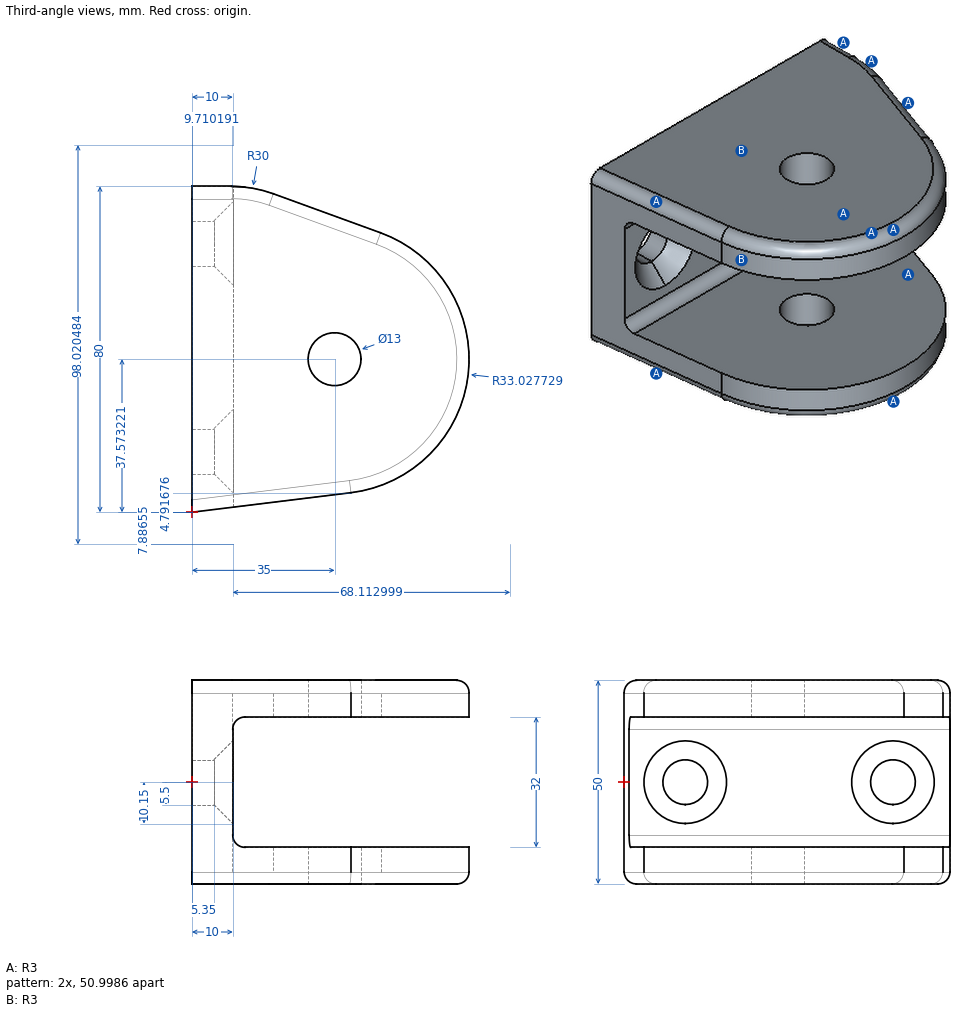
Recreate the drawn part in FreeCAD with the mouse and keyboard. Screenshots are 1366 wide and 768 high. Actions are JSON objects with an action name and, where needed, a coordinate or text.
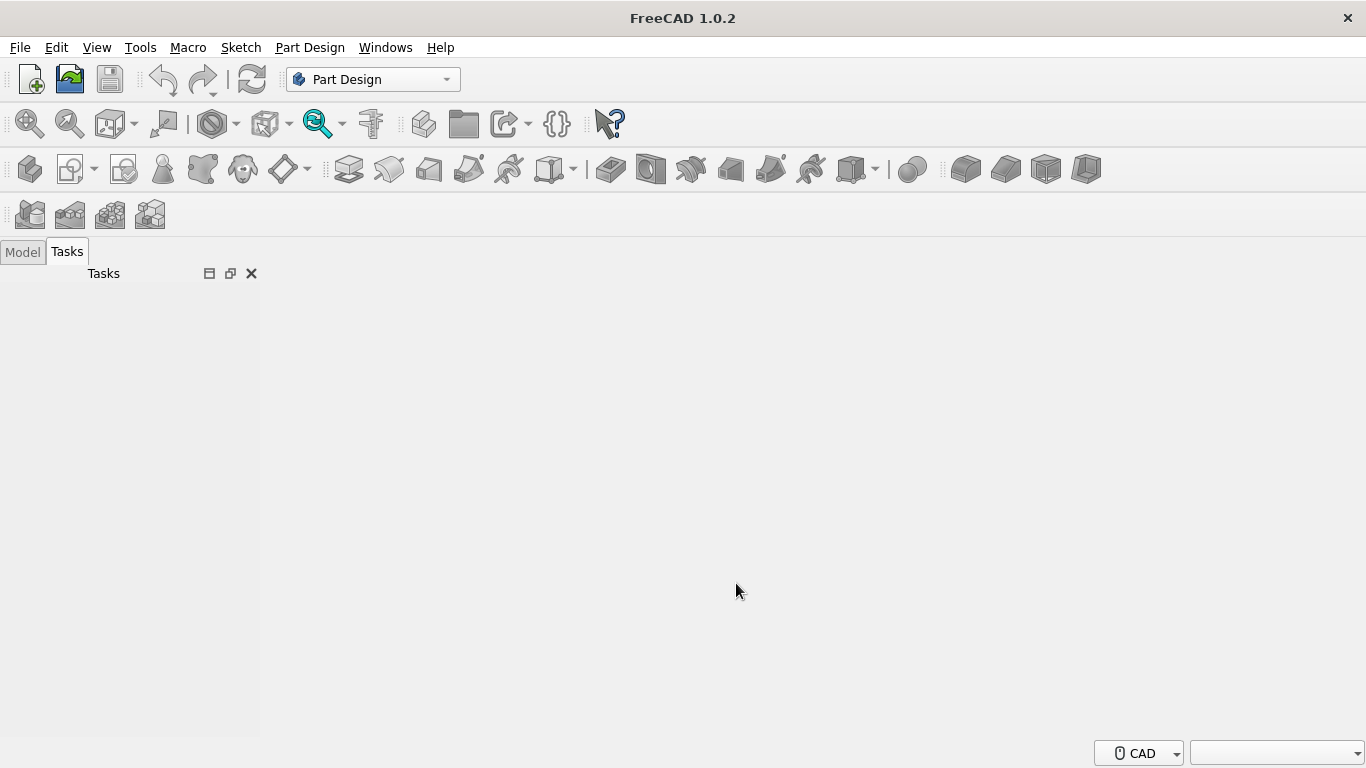
{"action": "left_click", "coordinate": [30, 80]}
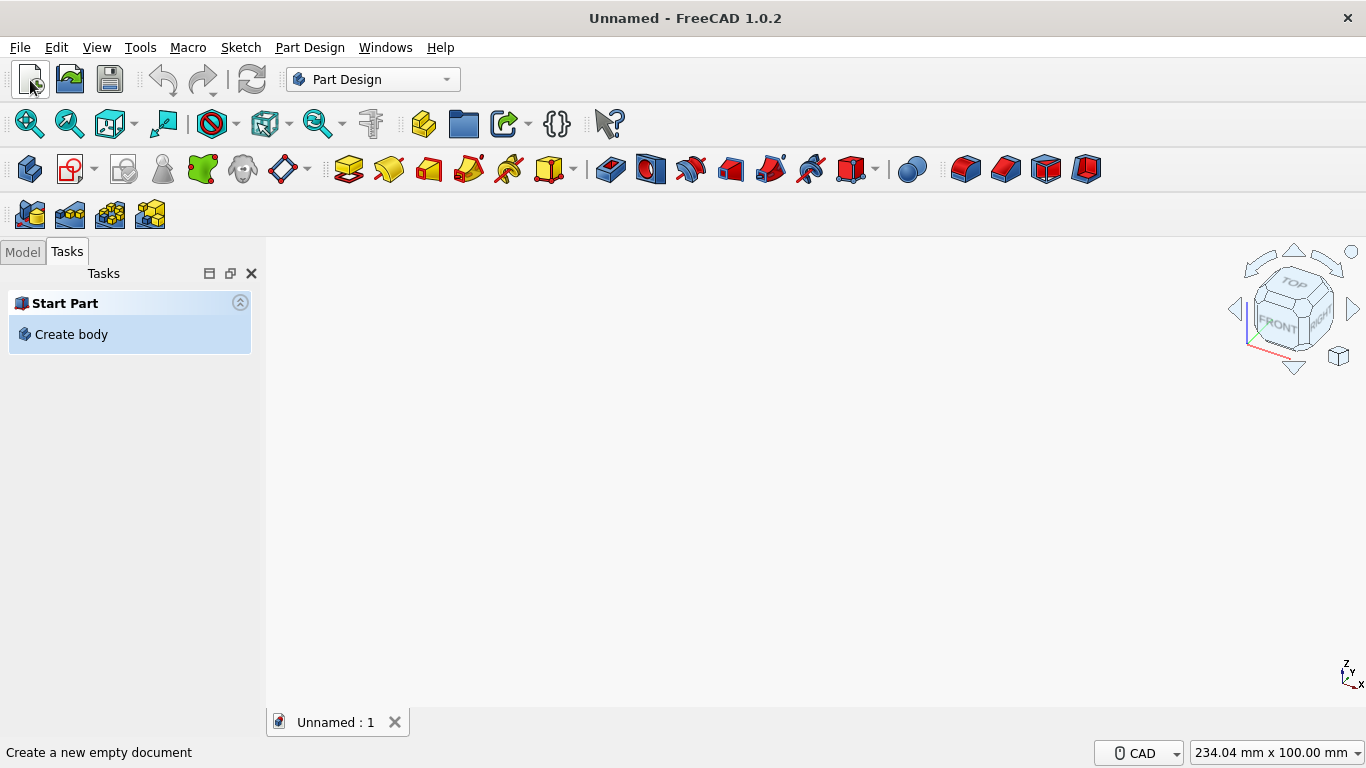
{"action": "left_click", "coordinate": [70, 170]}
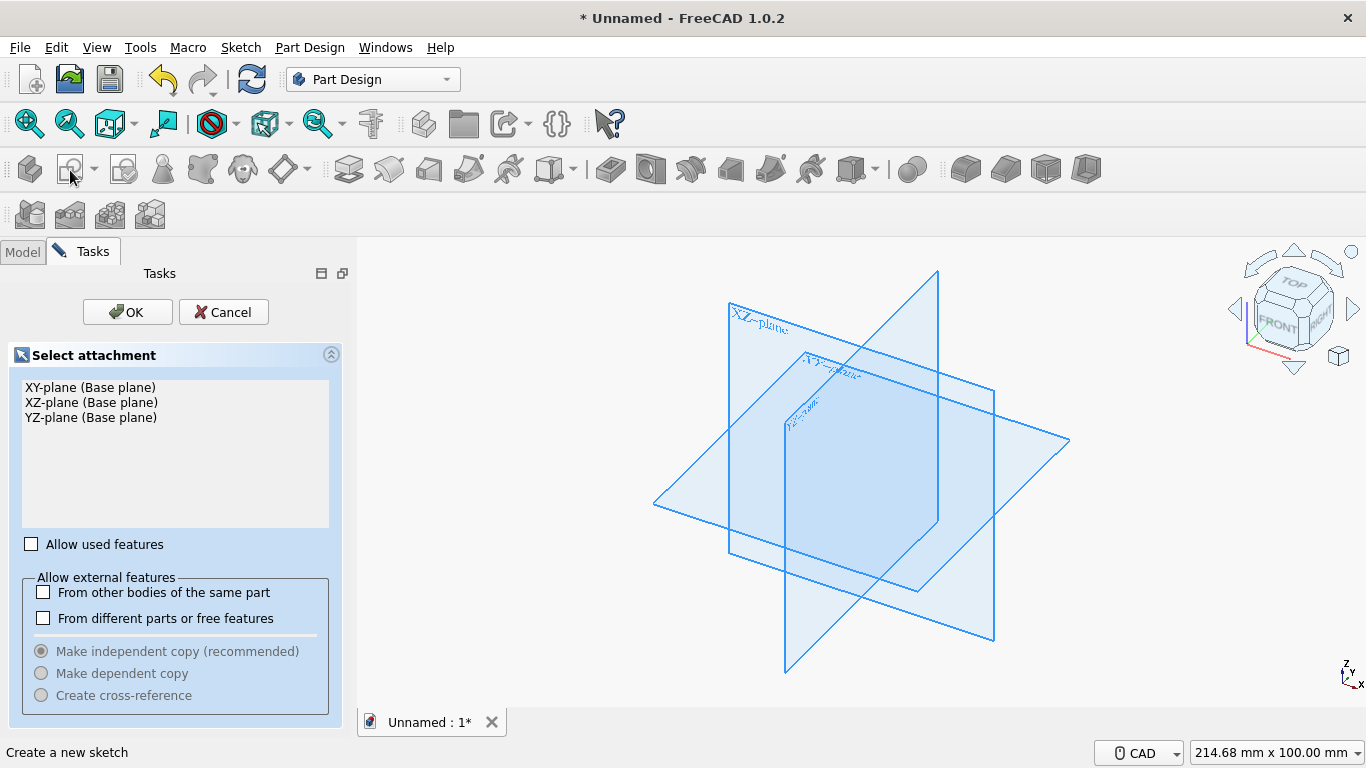
{"action": "left_click", "coordinate": [82, 388]}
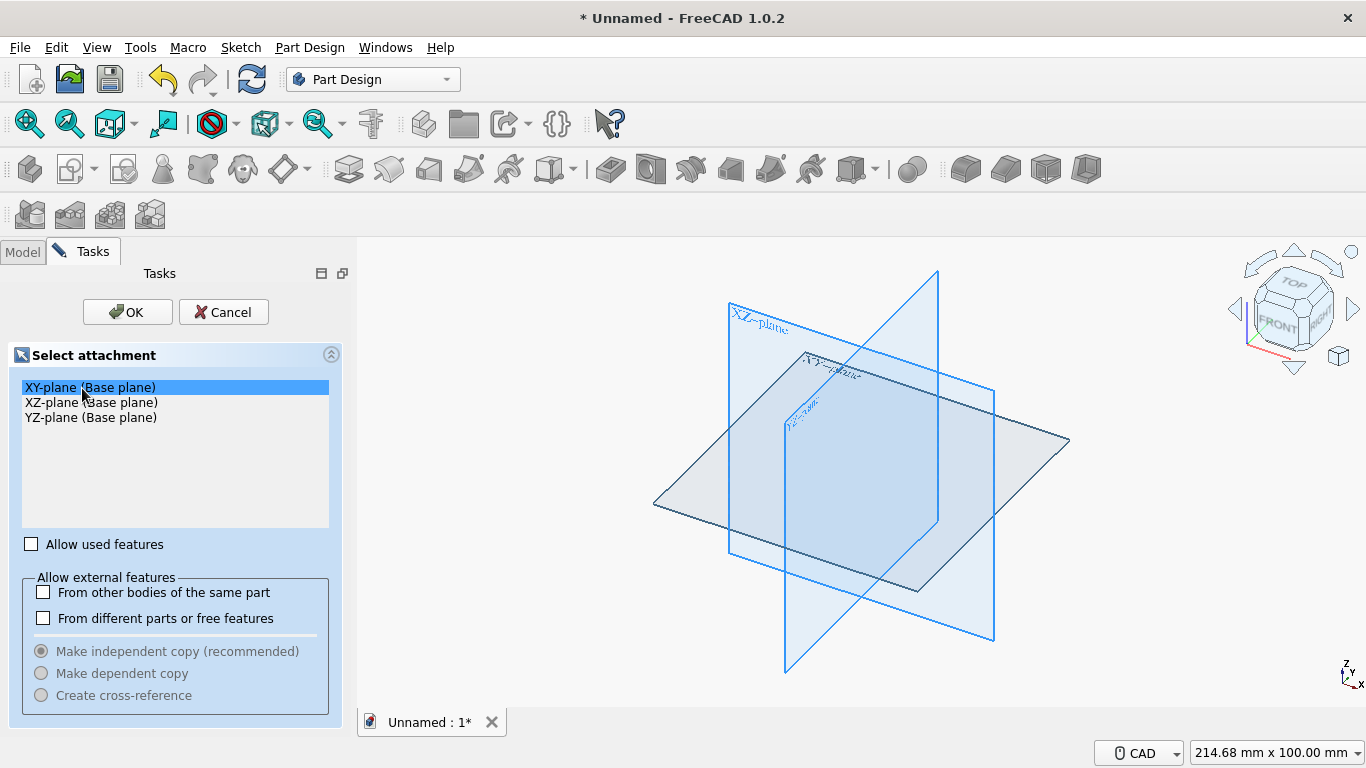
{"action": "left_click", "coordinate": [128, 312]}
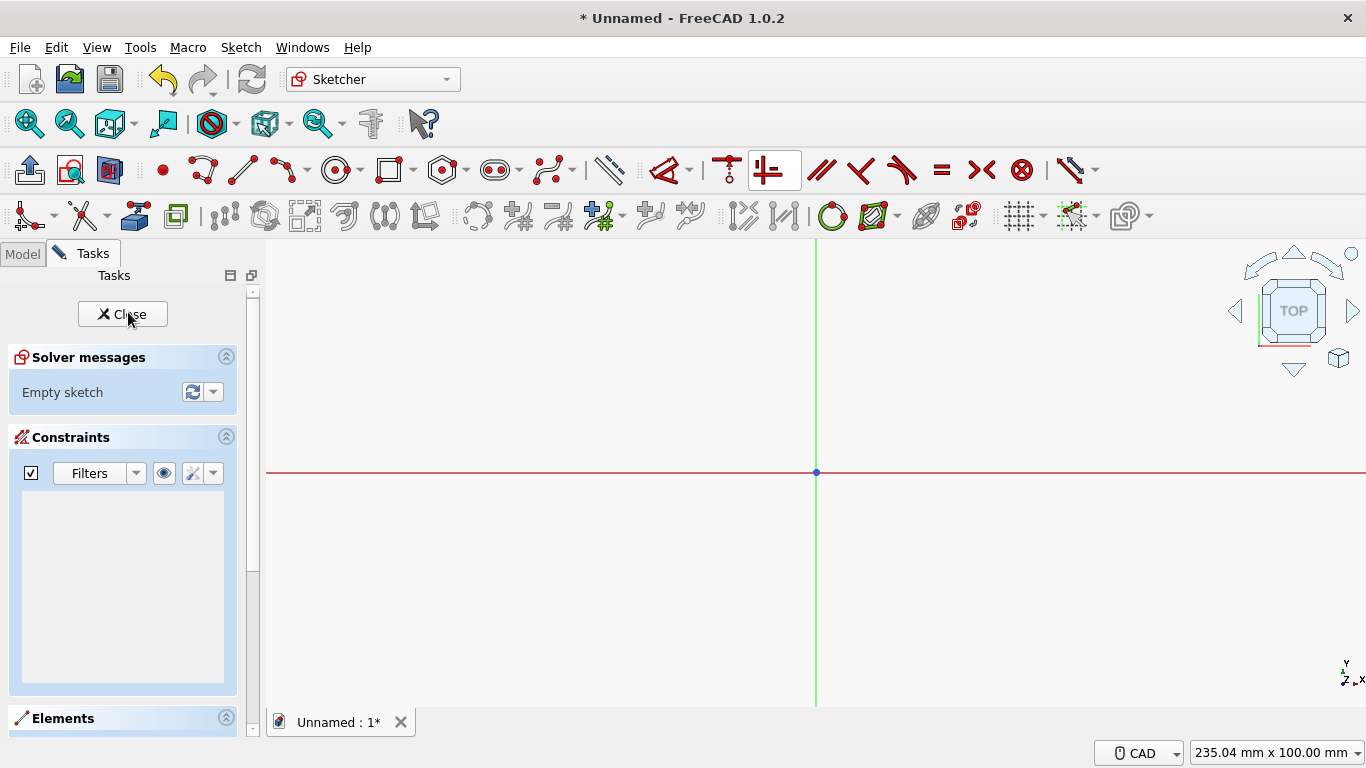
{"action": "scroll", "coordinate": [471, 679], "scroll_direction": "down", "scroll_amount": 3}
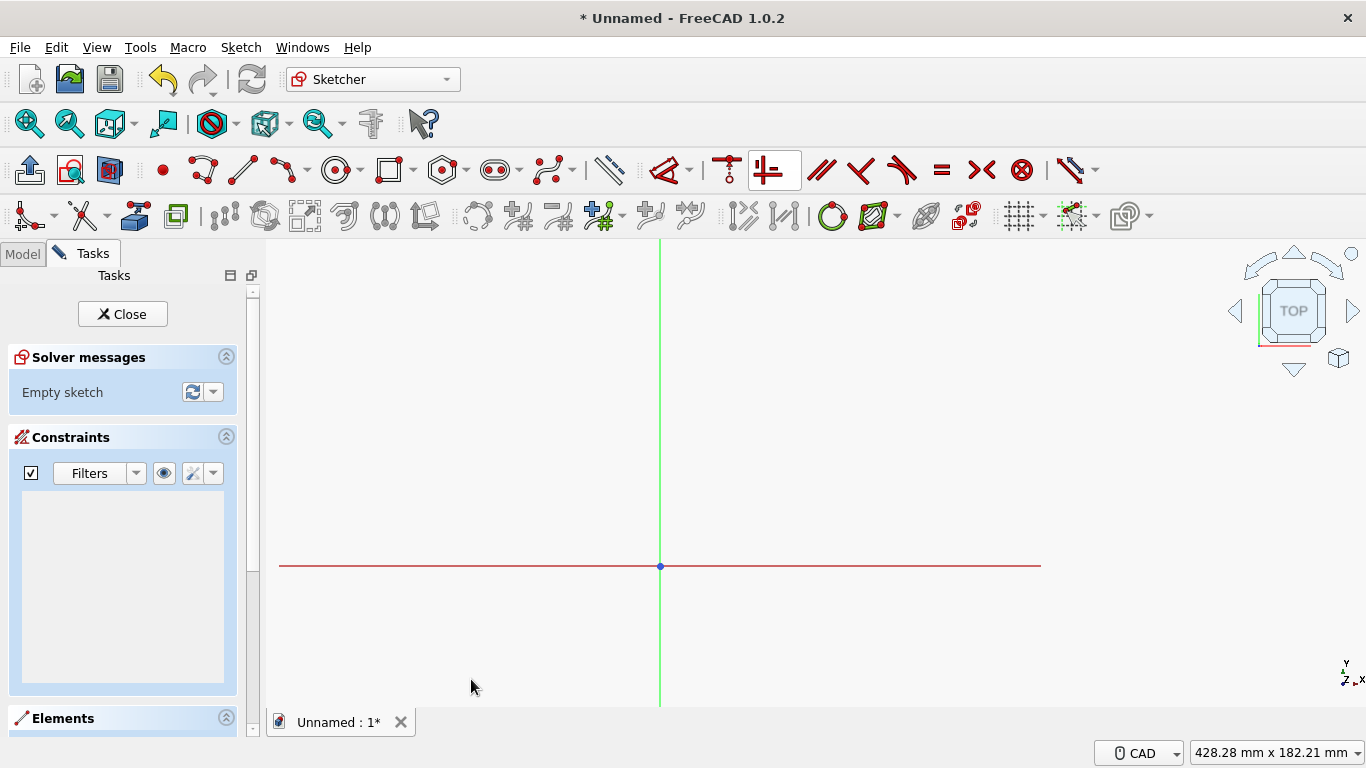
{"action": "scroll", "coordinate": [748, 445], "scroll_direction": "up", "scroll_amount": 2}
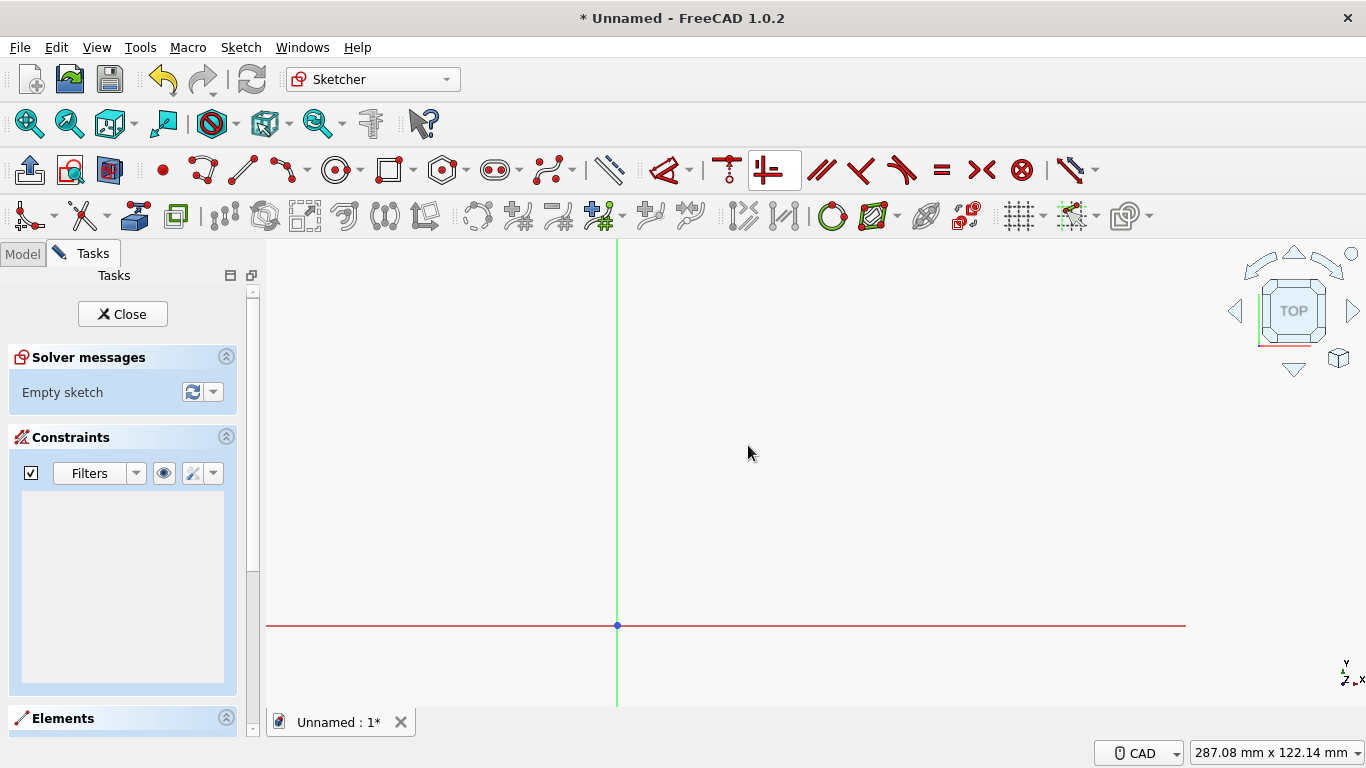
{"action": "left_click", "coordinate": [244, 170]}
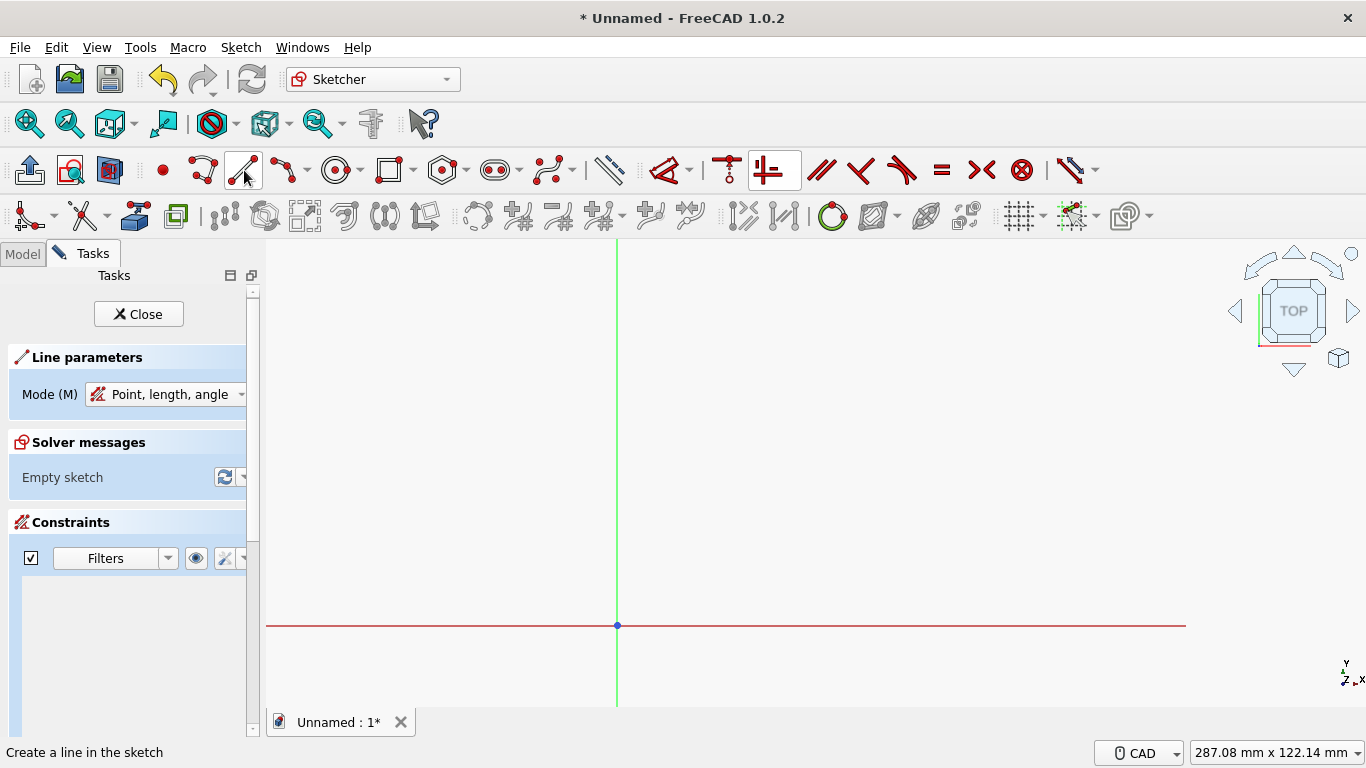
{"action": "left_click", "coordinate": [795, 363]}
{"action": "left_click", "coordinate": [694, 326]}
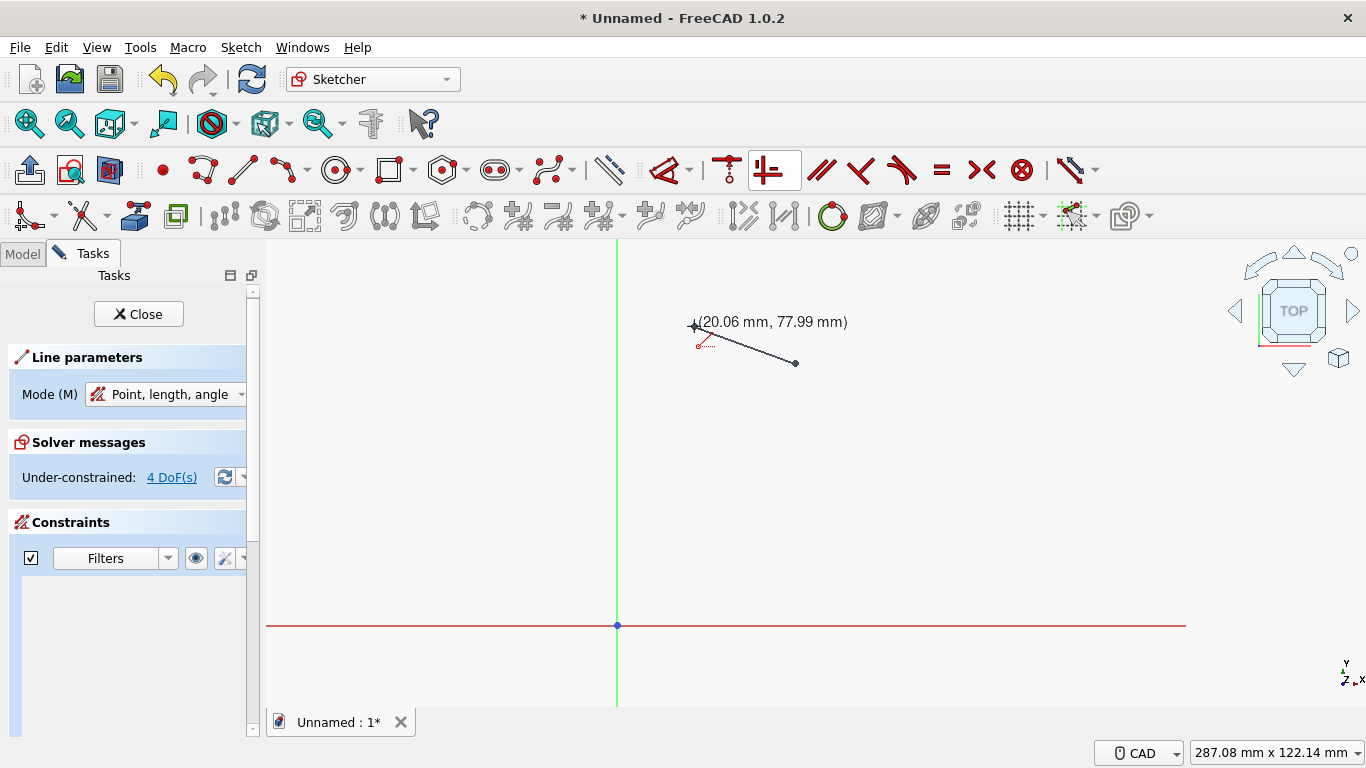
{"action": "left_click", "coordinate": [204, 170]}